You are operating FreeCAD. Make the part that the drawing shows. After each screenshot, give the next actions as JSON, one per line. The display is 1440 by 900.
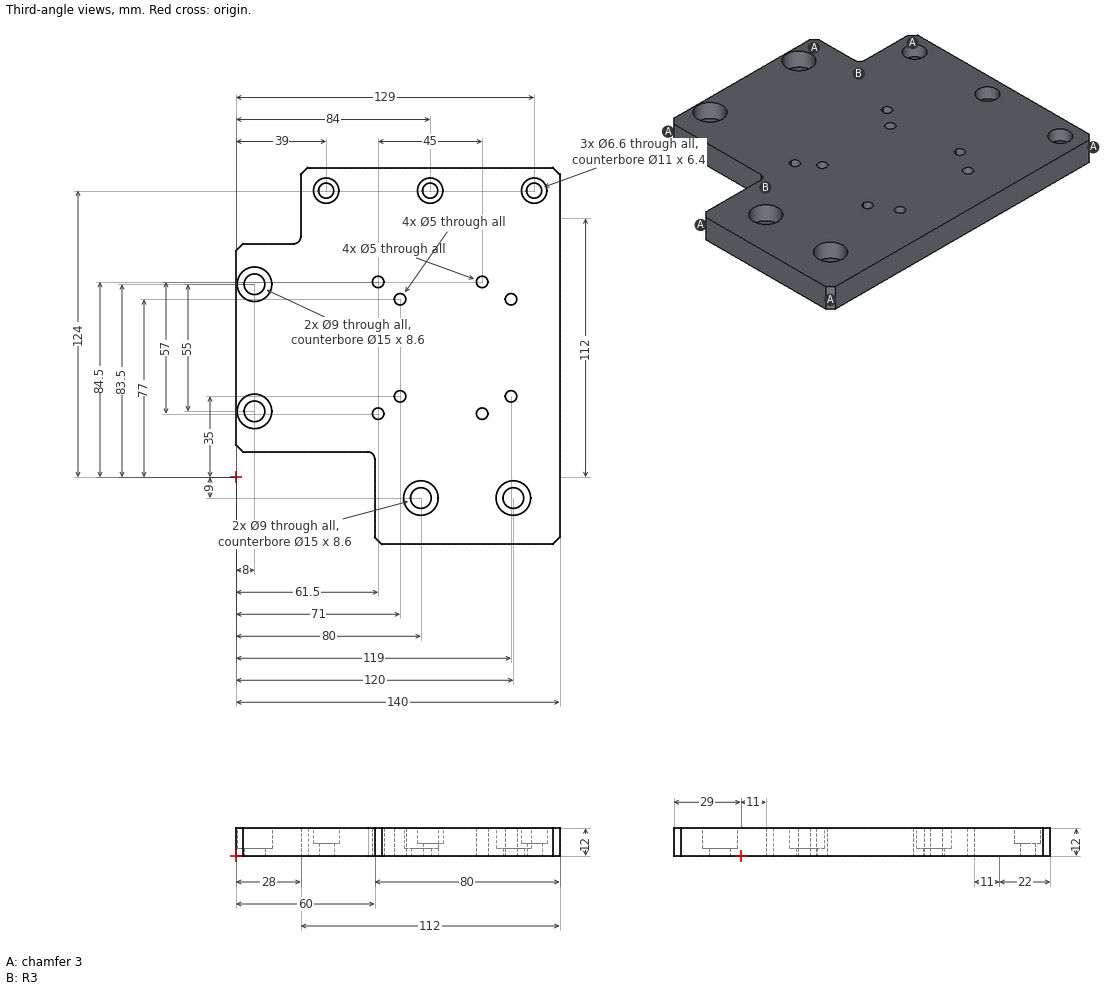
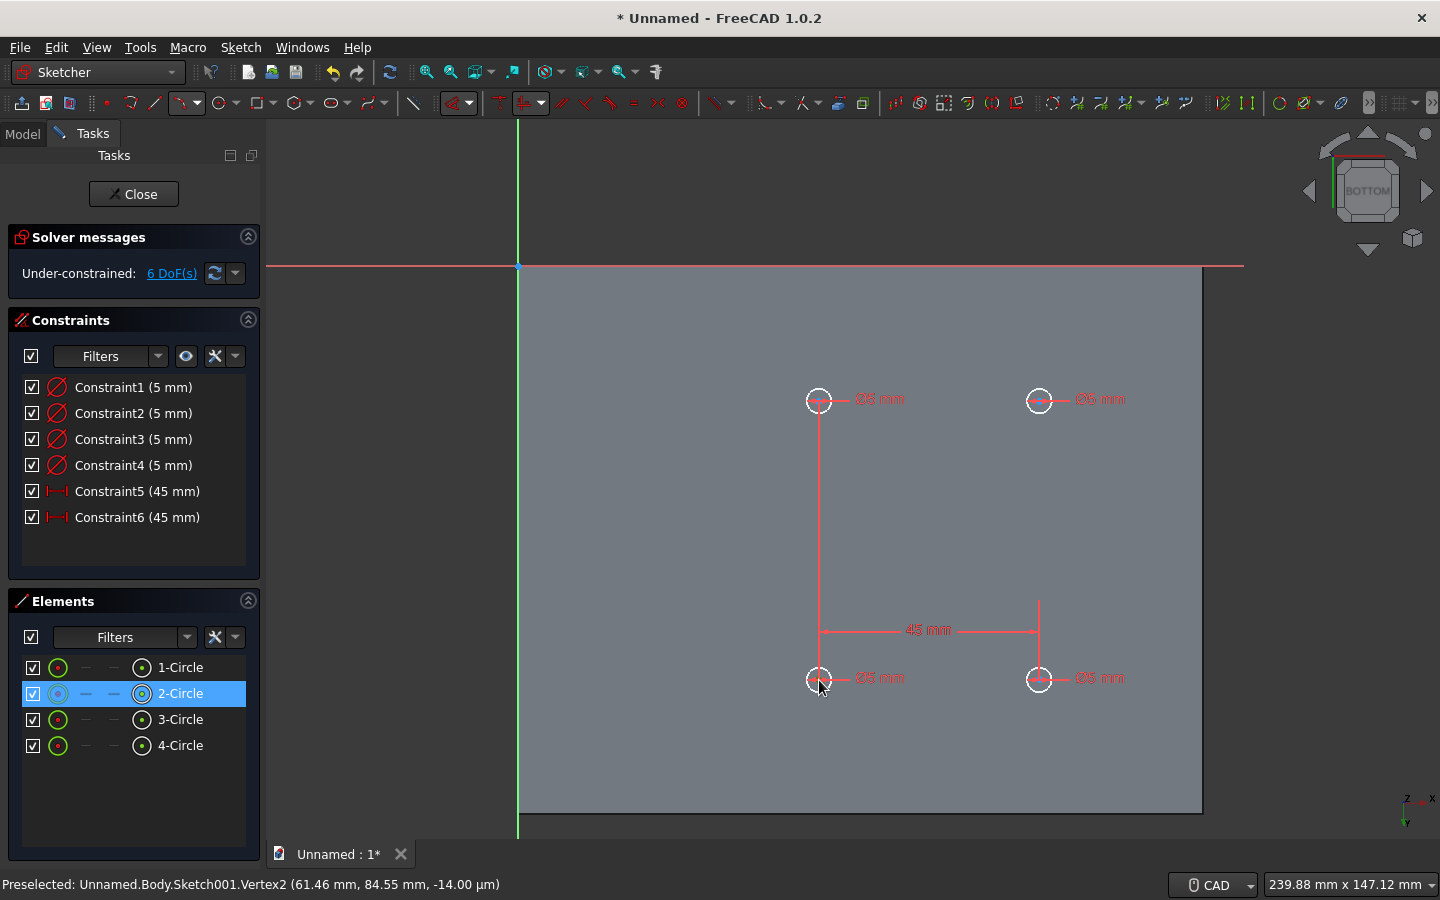
{"action": "left_click", "coordinate": [819, 401]}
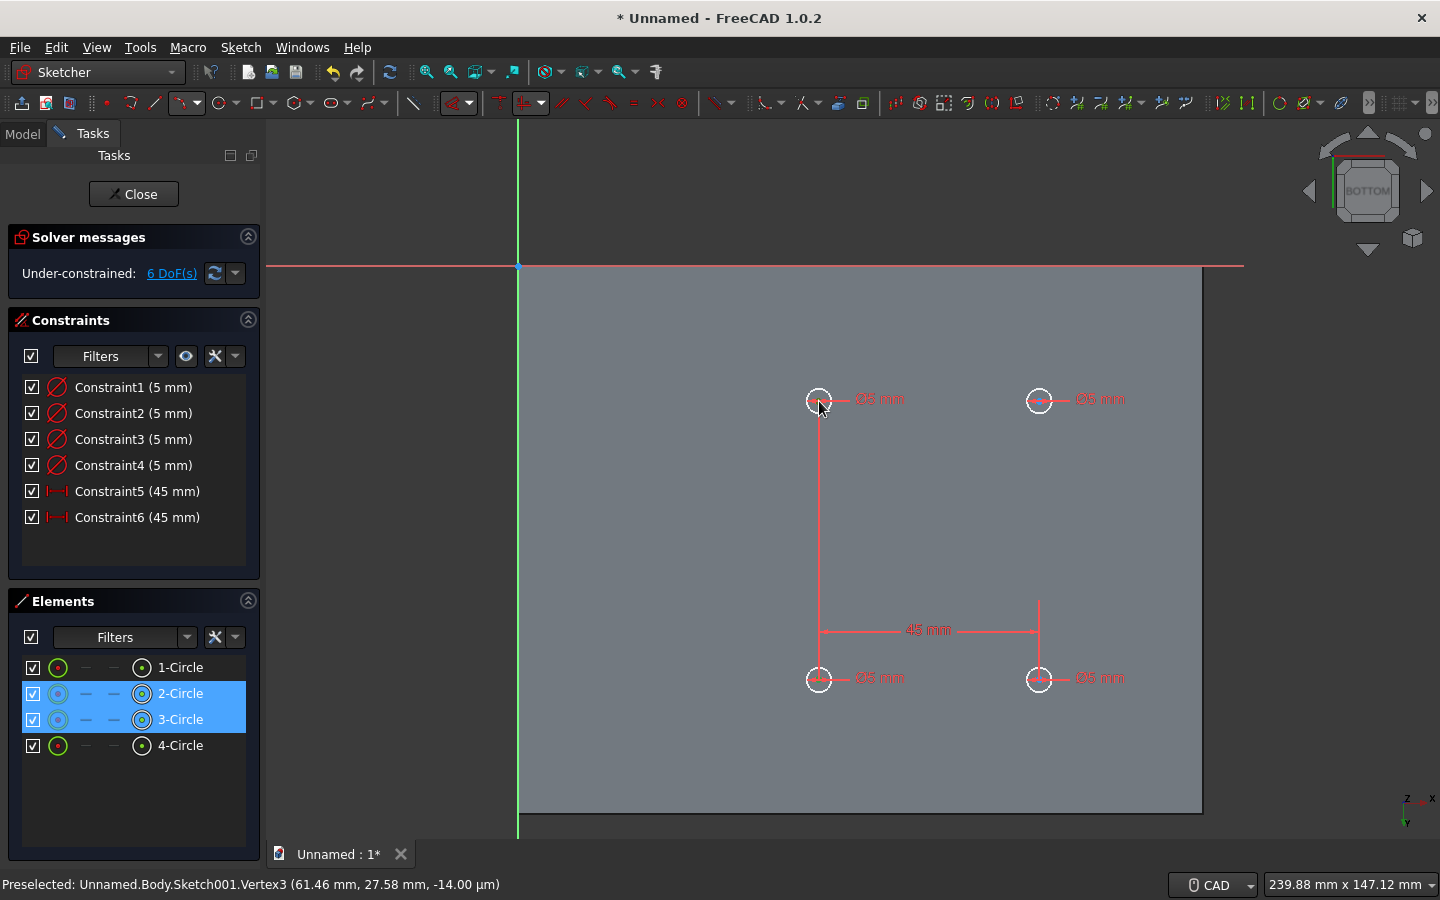
{"action": "key", "text": "i"}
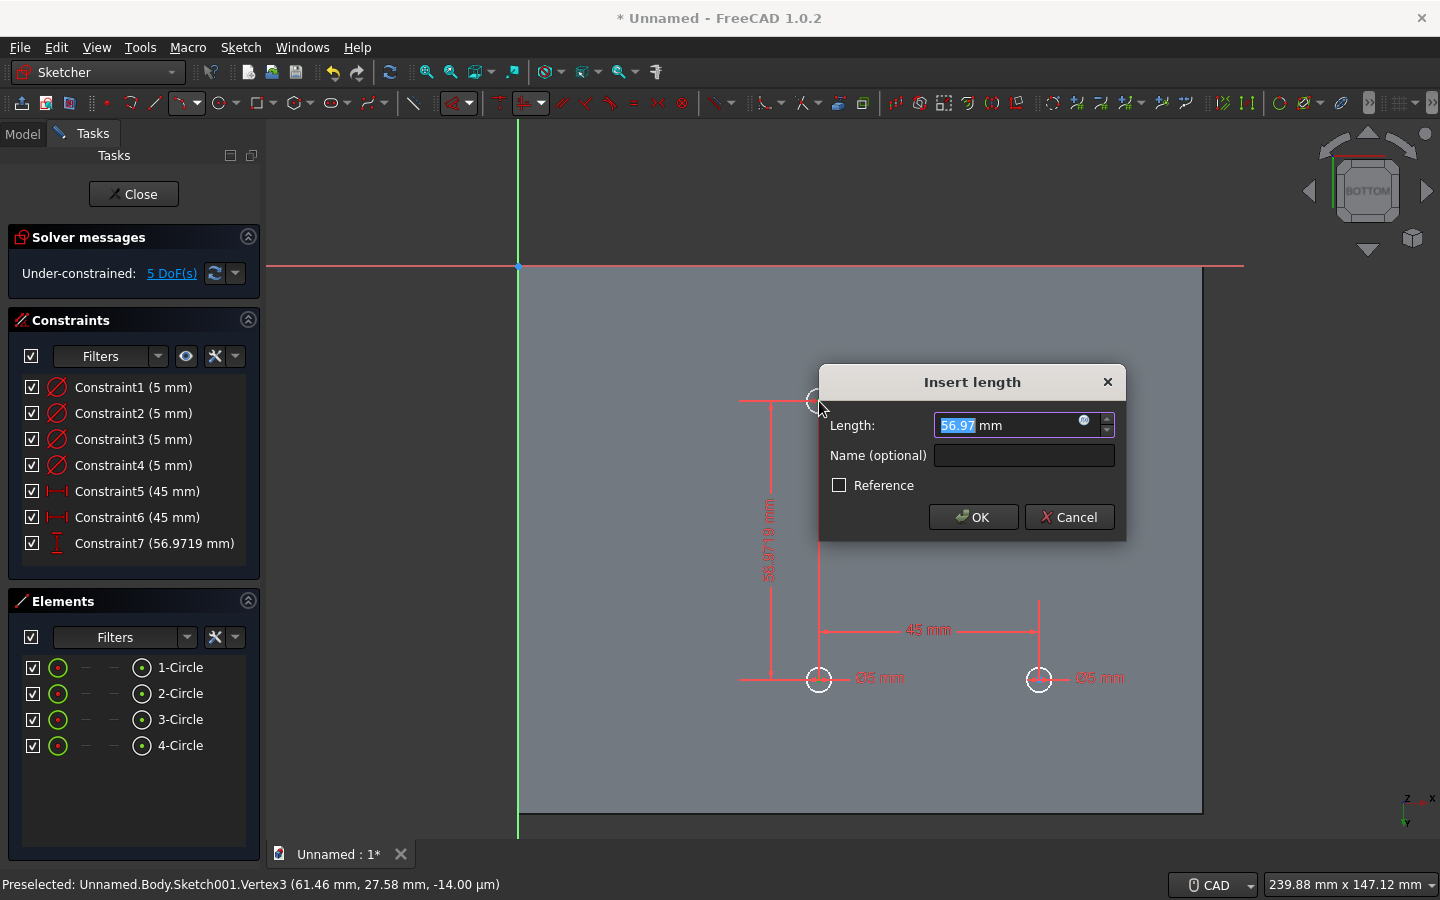
{"action": "type", "text": "57"}
{"action": "key", "text": "Return"}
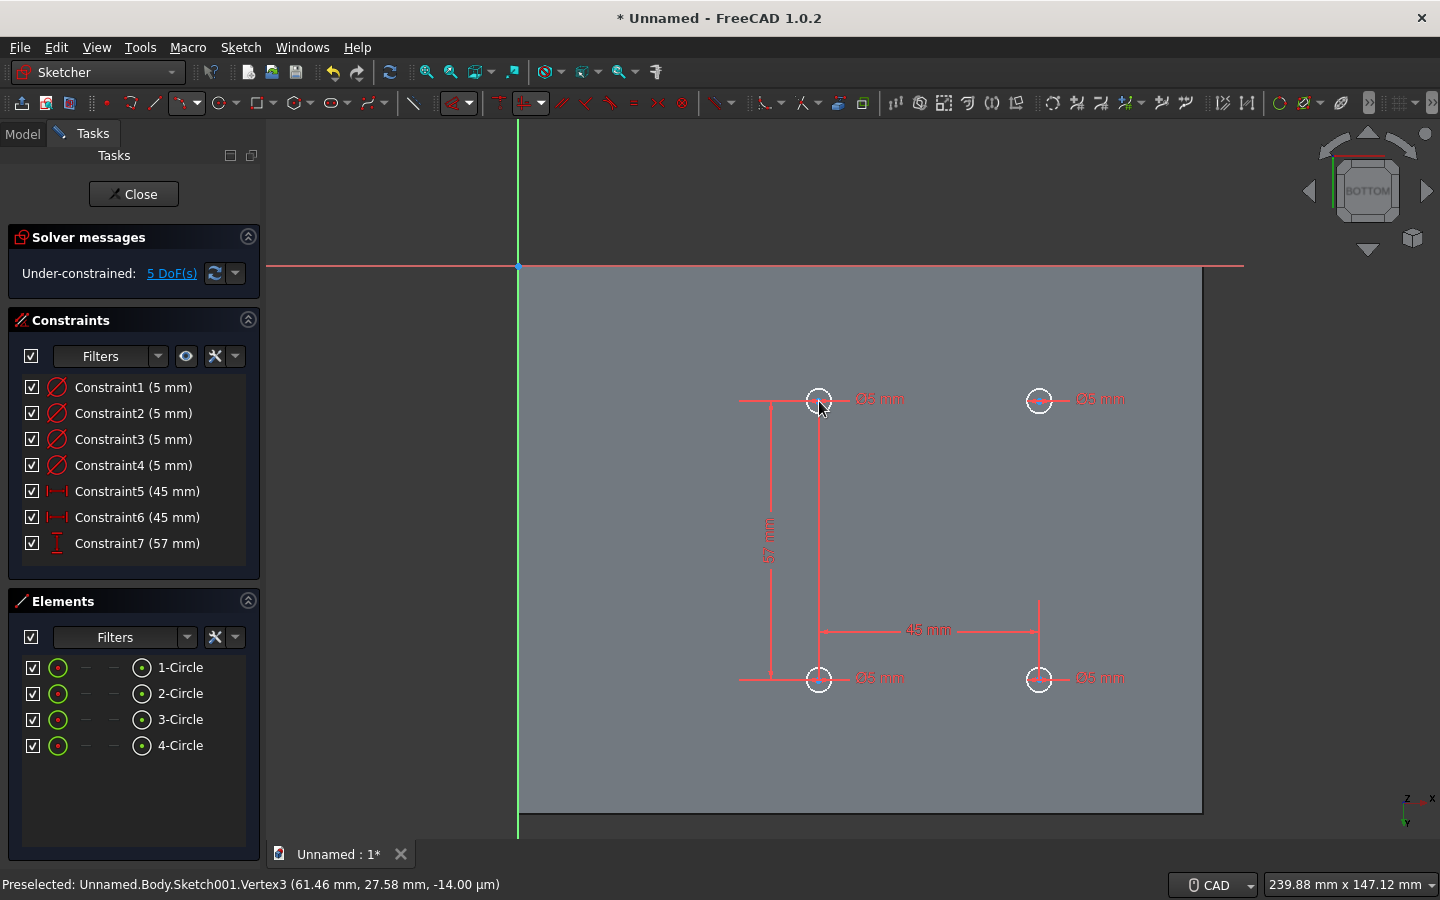
{"action": "left_click", "coordinate": [1039, 680]}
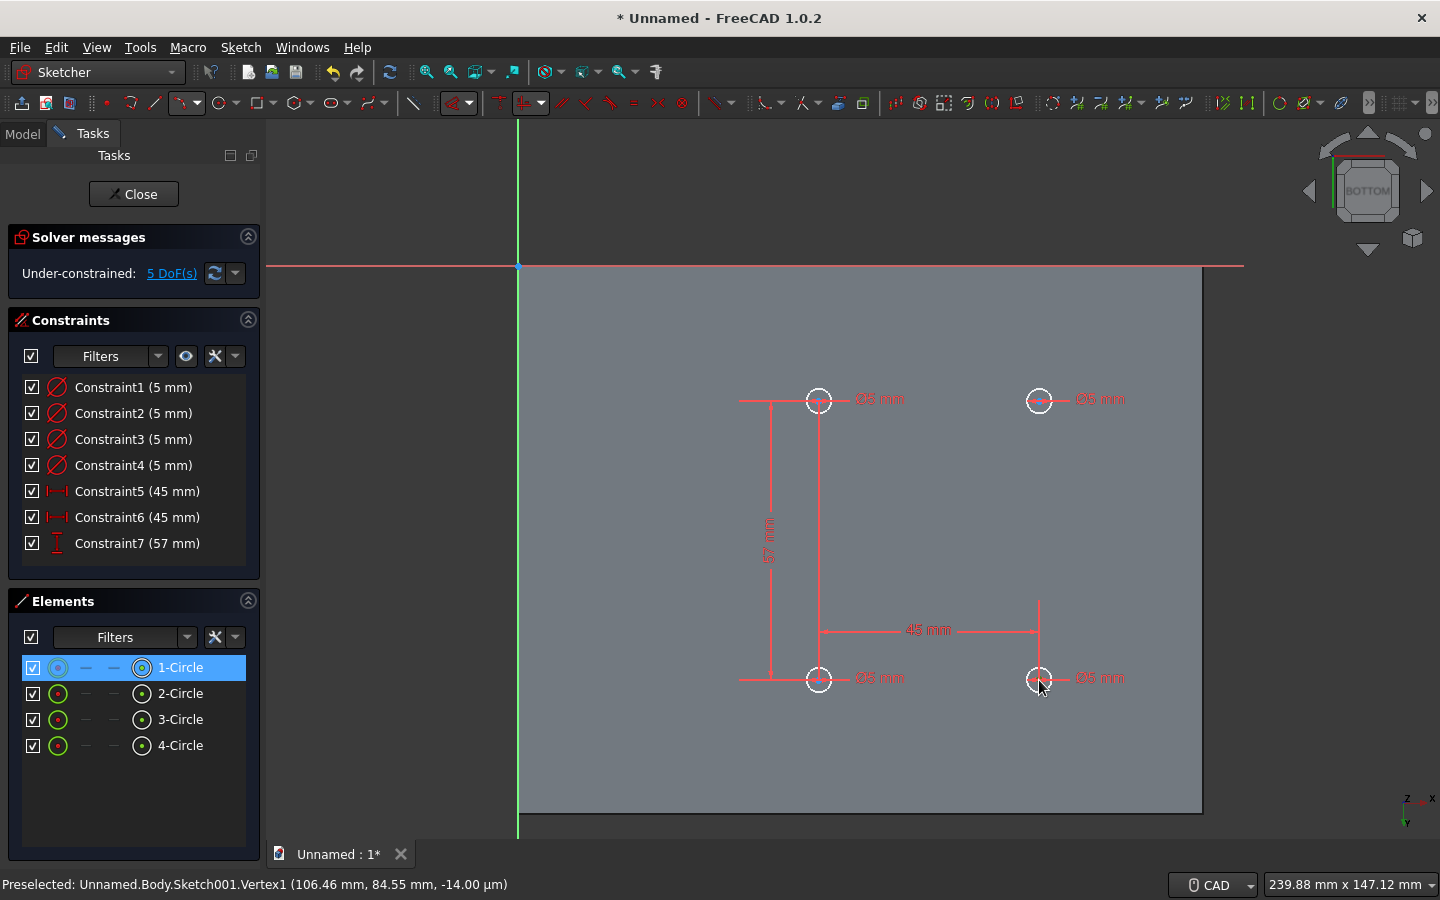
{"action": "left_click", "coordinate": [819, 401]}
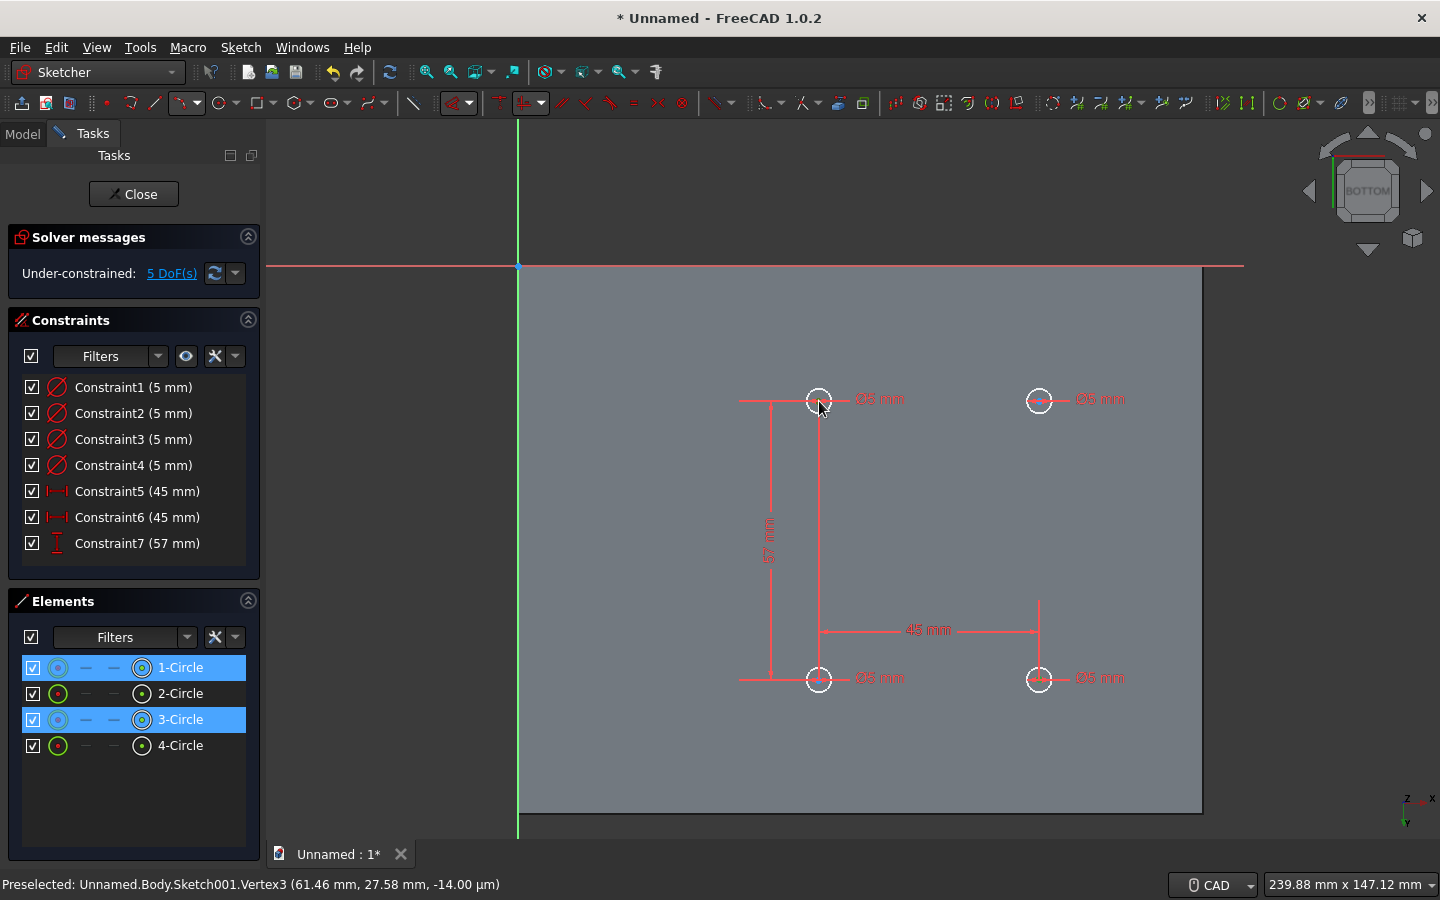
{"action": "key", "text": "i"}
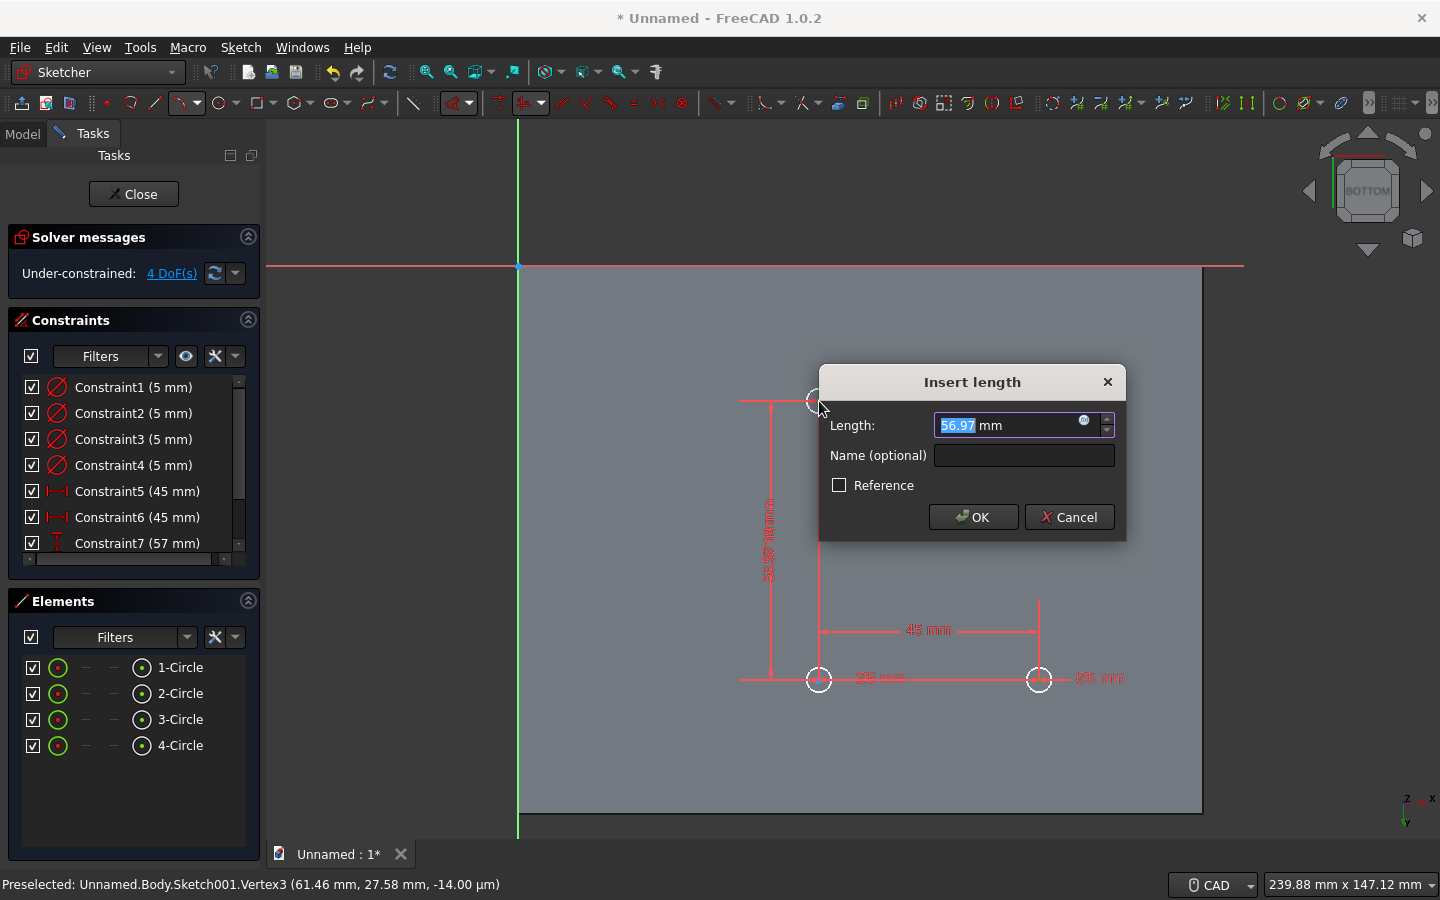
{"action": "type", "text": "57"}
{"action": "key", "text": "Return"}